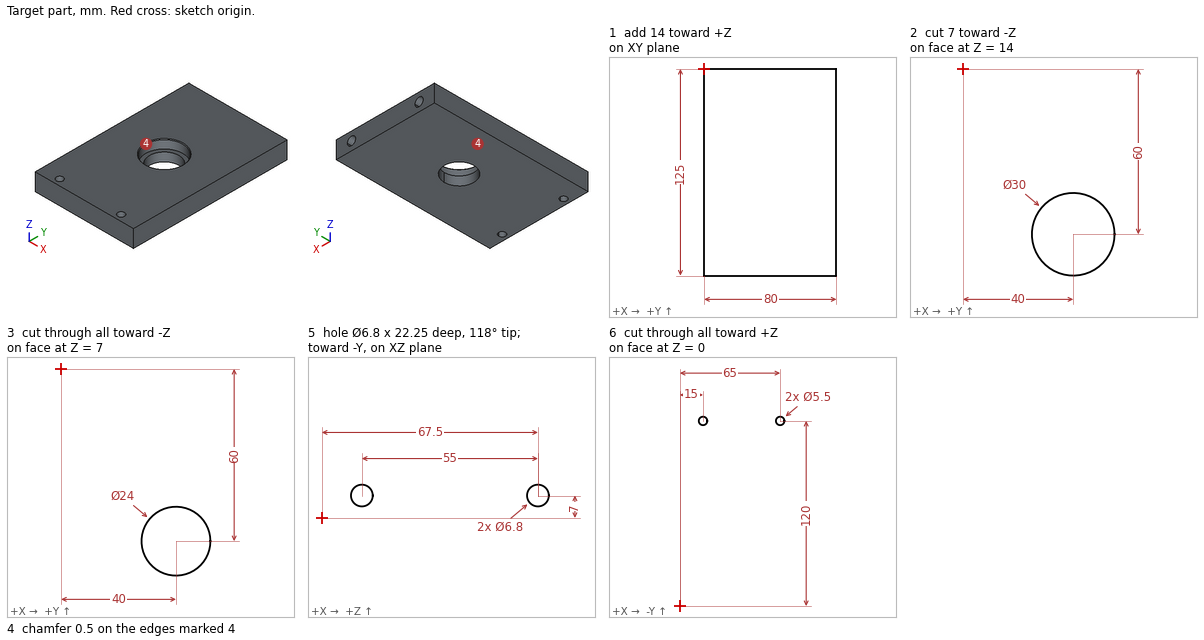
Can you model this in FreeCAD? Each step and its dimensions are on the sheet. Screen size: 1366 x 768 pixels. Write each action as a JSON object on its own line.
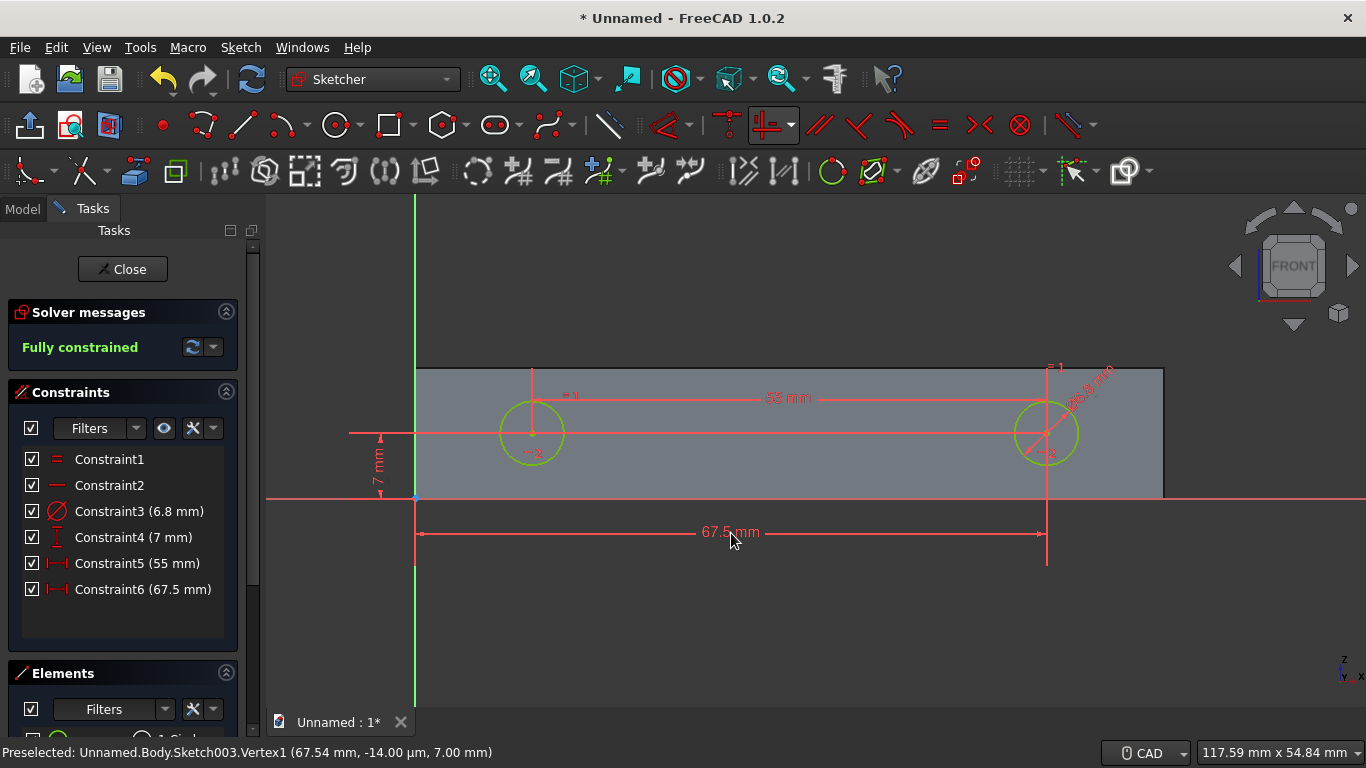
{"action": "left_click", "coordinate": [123, 269]}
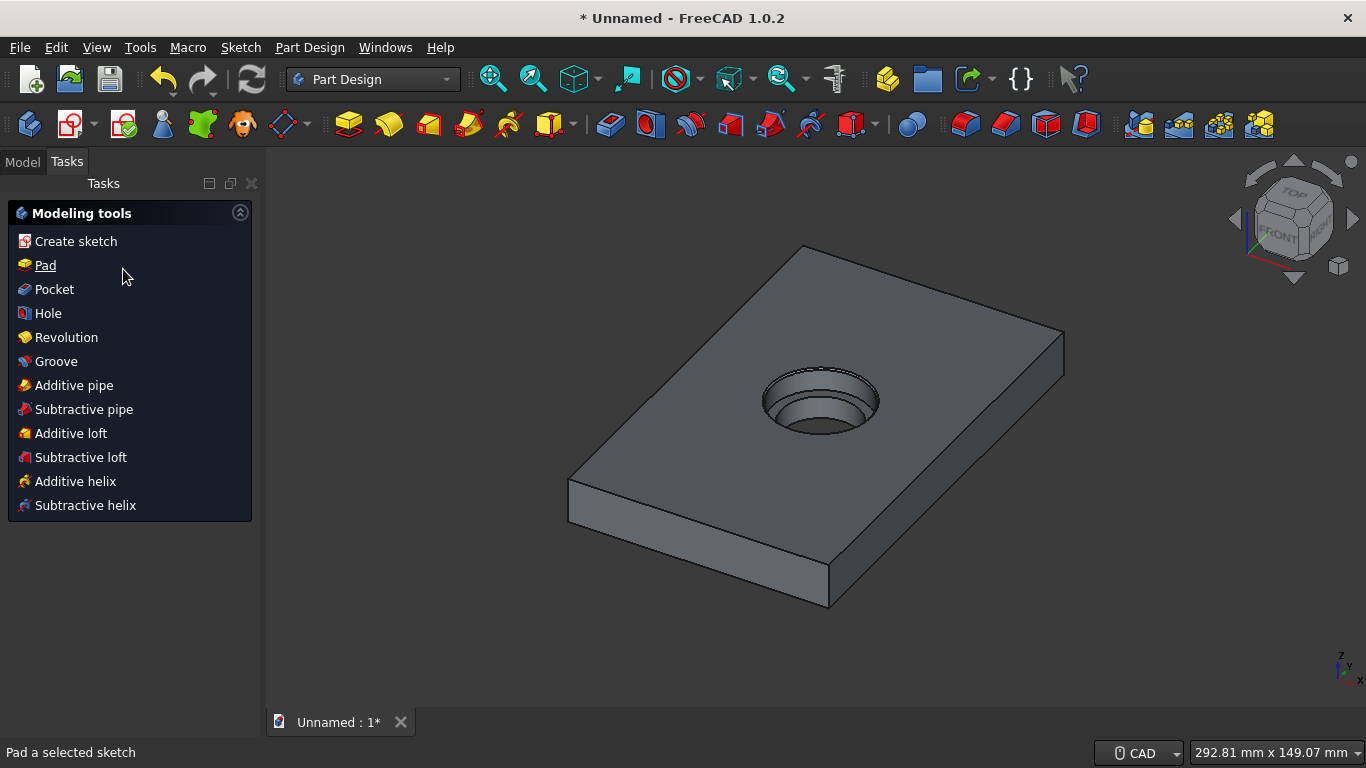
{"action": "left_click", "coordinate": [652, 124]}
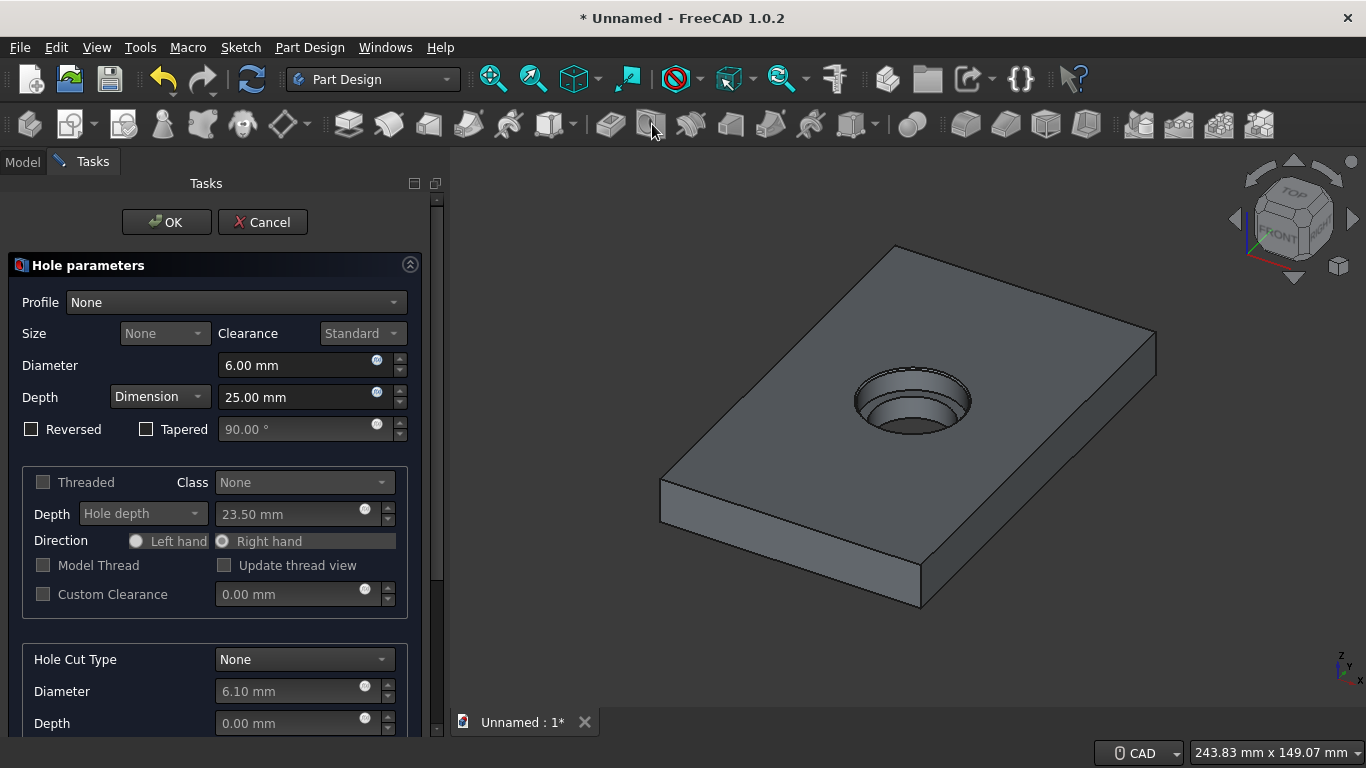
{"action": "triple_click", "coordinate": [305, 365]}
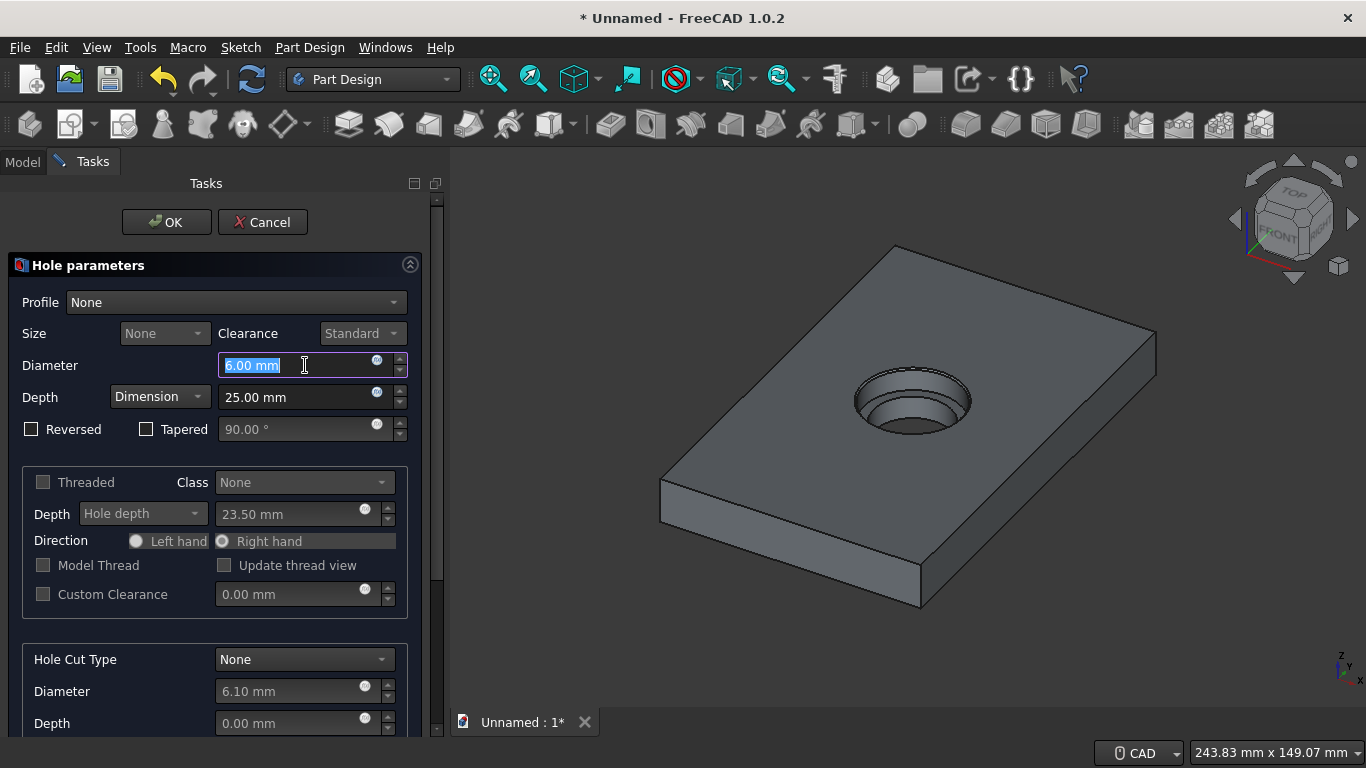
{"action": "type", "text": "6.8"}
{"action": "key", "text": "Tab"}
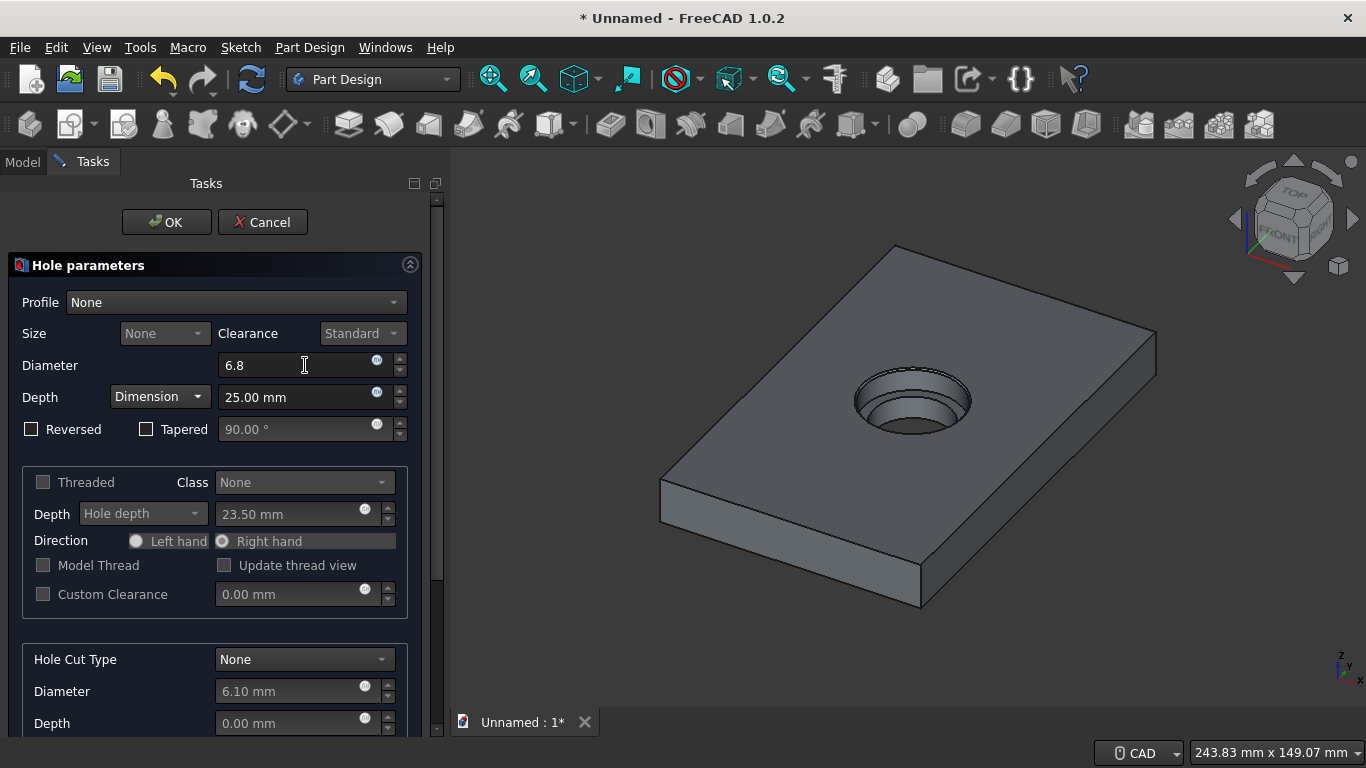
{"action": "triple_click", "coordinate": [305, 397]}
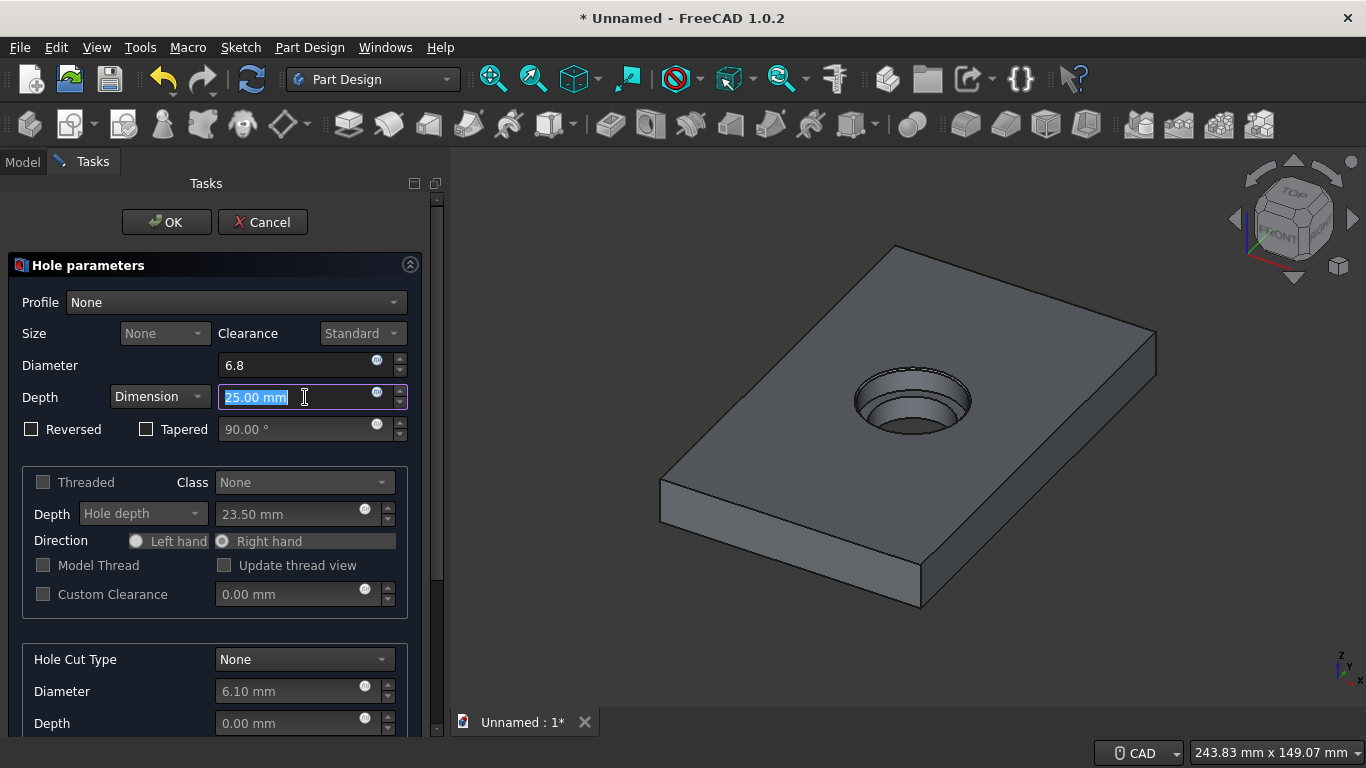
{"action": "type", "text": "22.25"}
{"action": "key", "text": "Tab"}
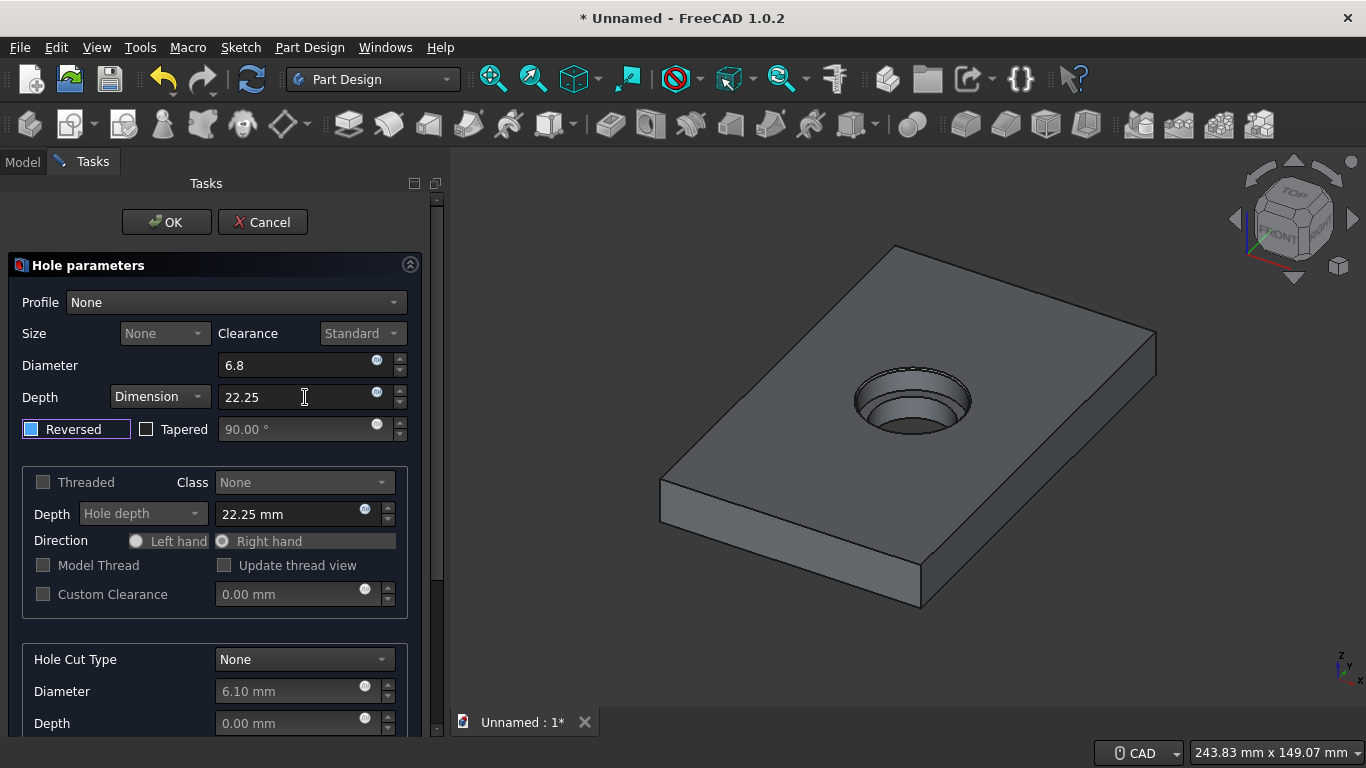
{"action": "left_click", "coordinate": [30, 429]}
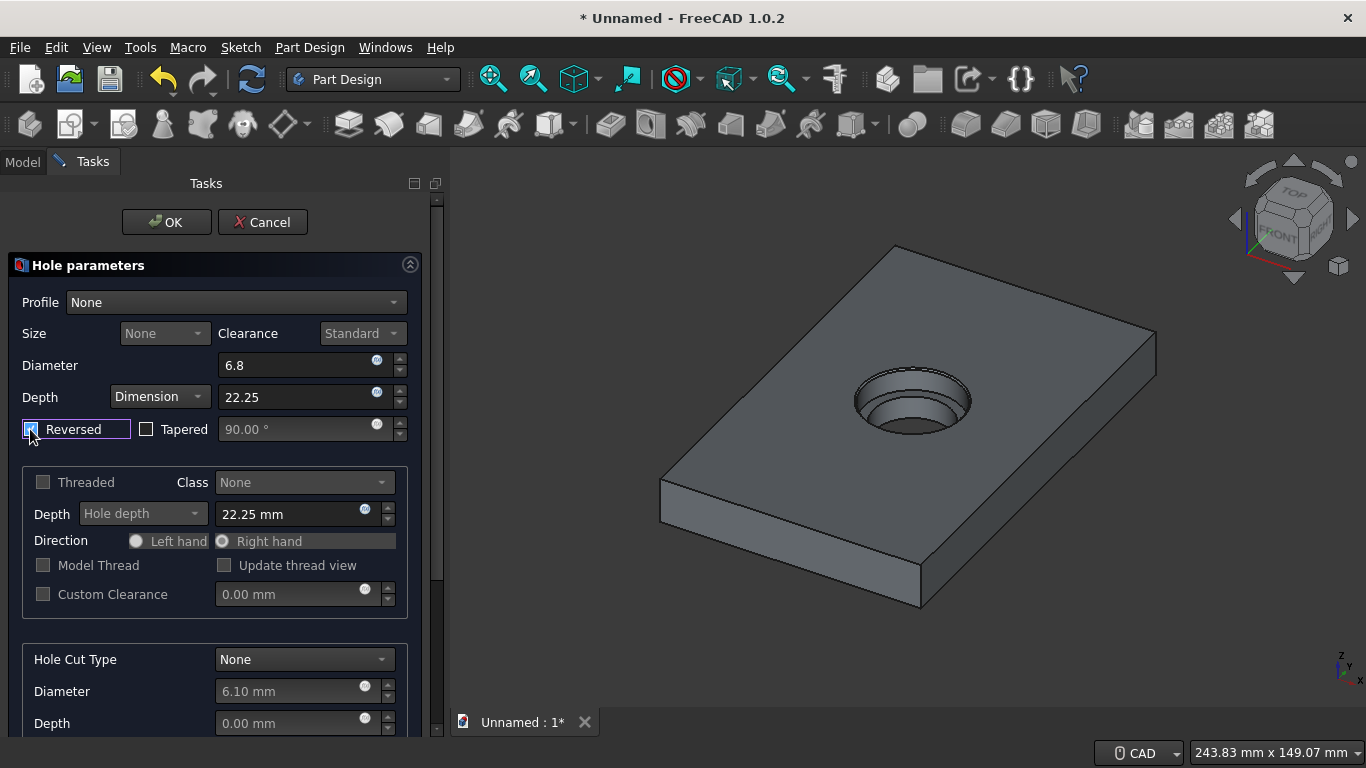
{"action": "left_click", "coordinate": [167, 222]}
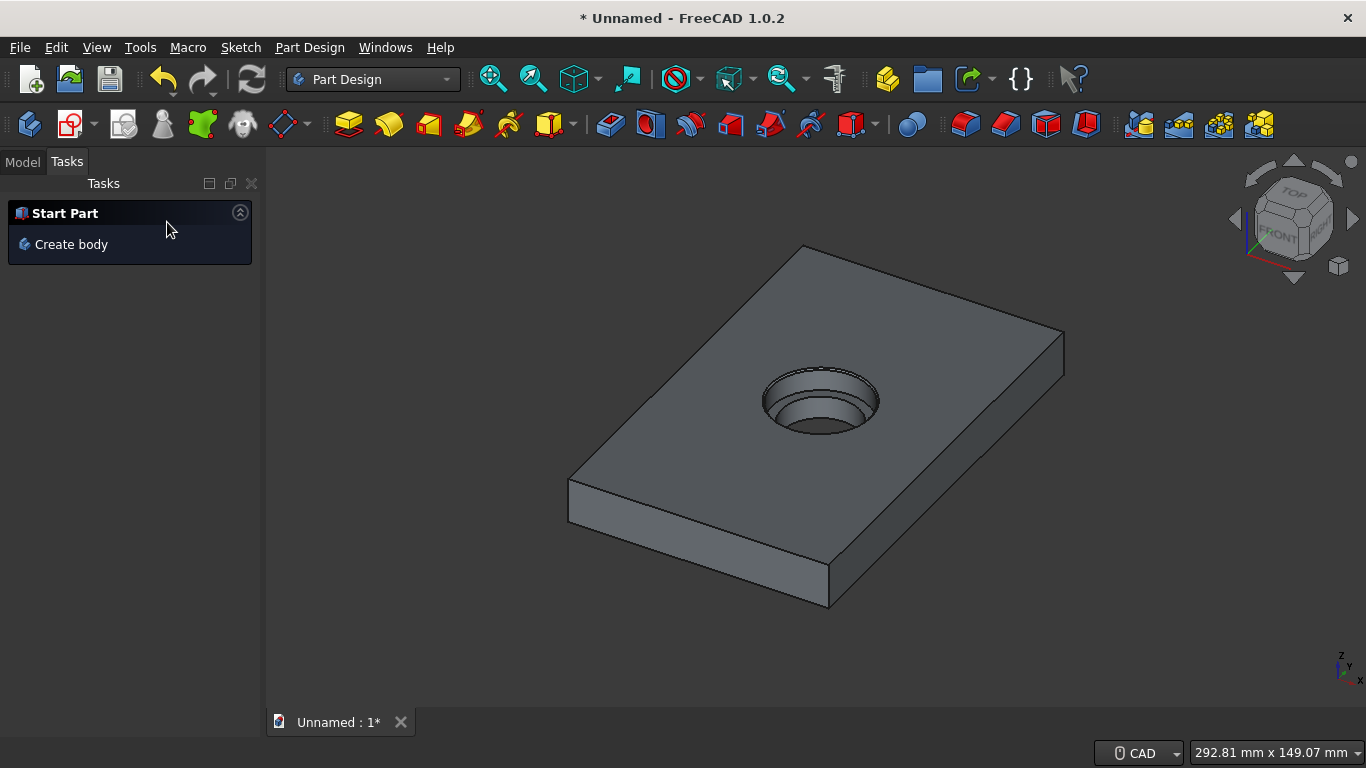
{"action": "key", "text": "5"}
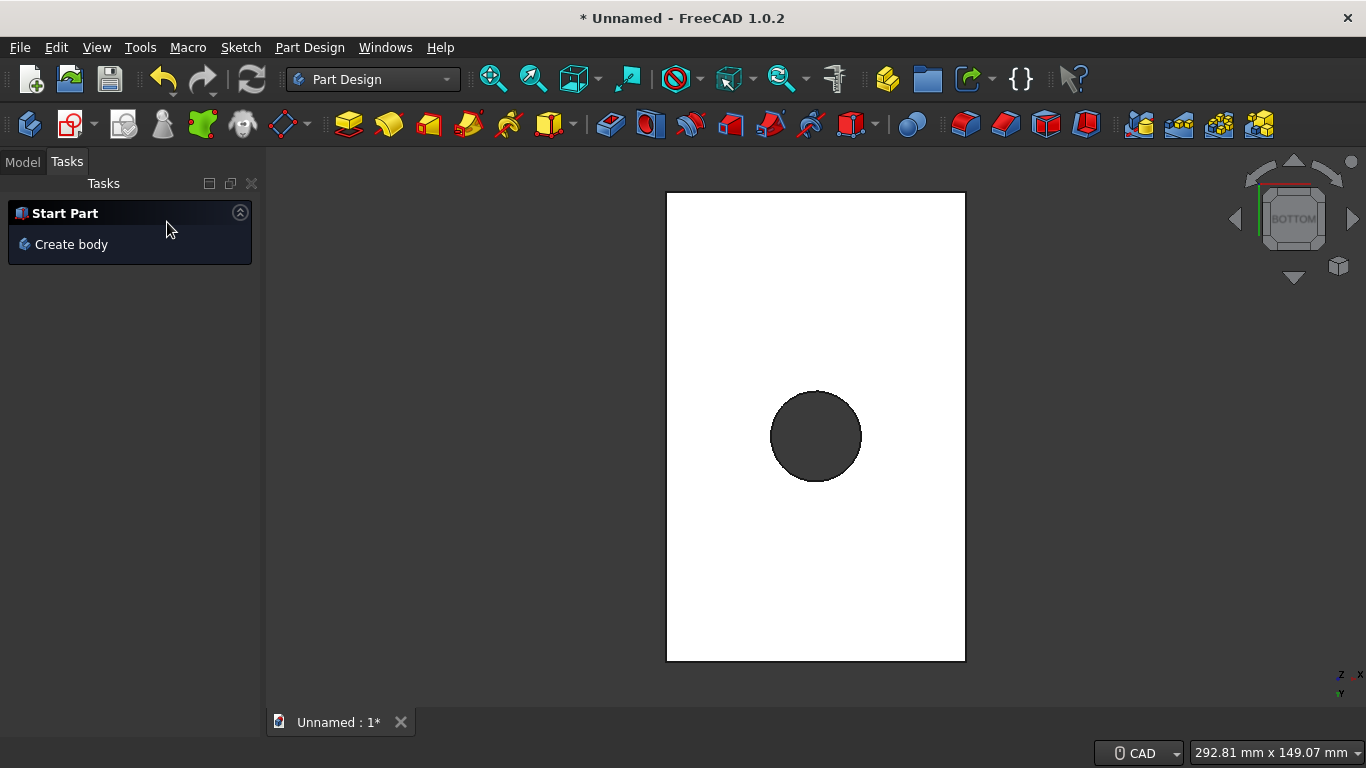
{"action": "left_click", "coordinate": [859, 292]}